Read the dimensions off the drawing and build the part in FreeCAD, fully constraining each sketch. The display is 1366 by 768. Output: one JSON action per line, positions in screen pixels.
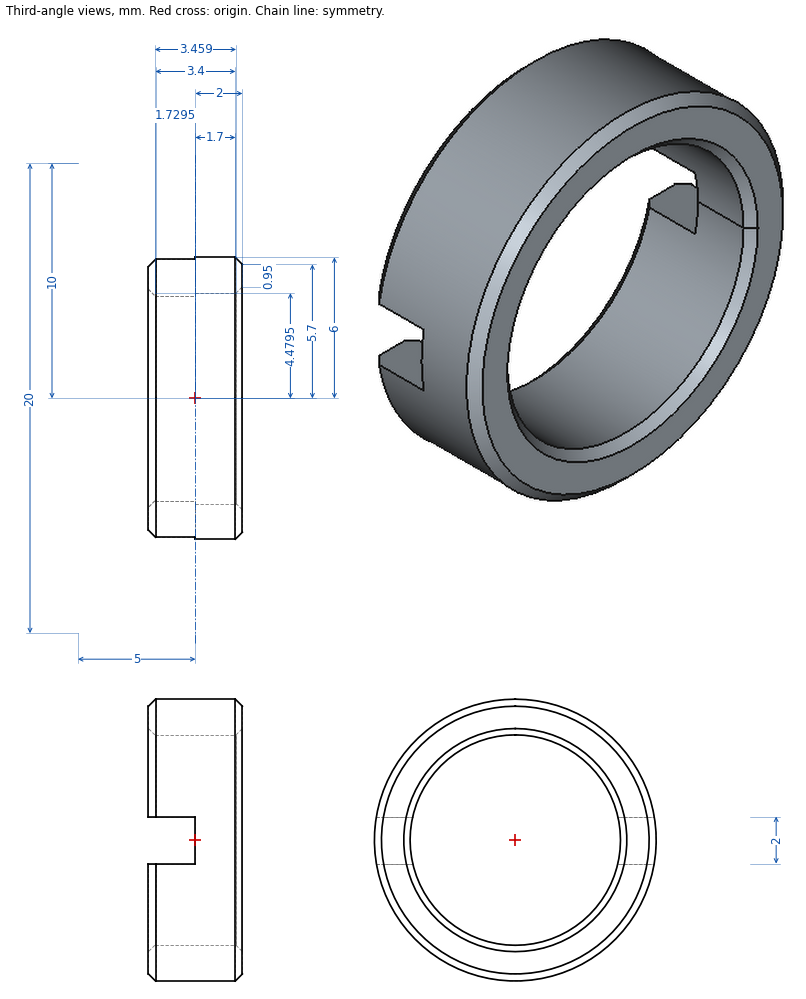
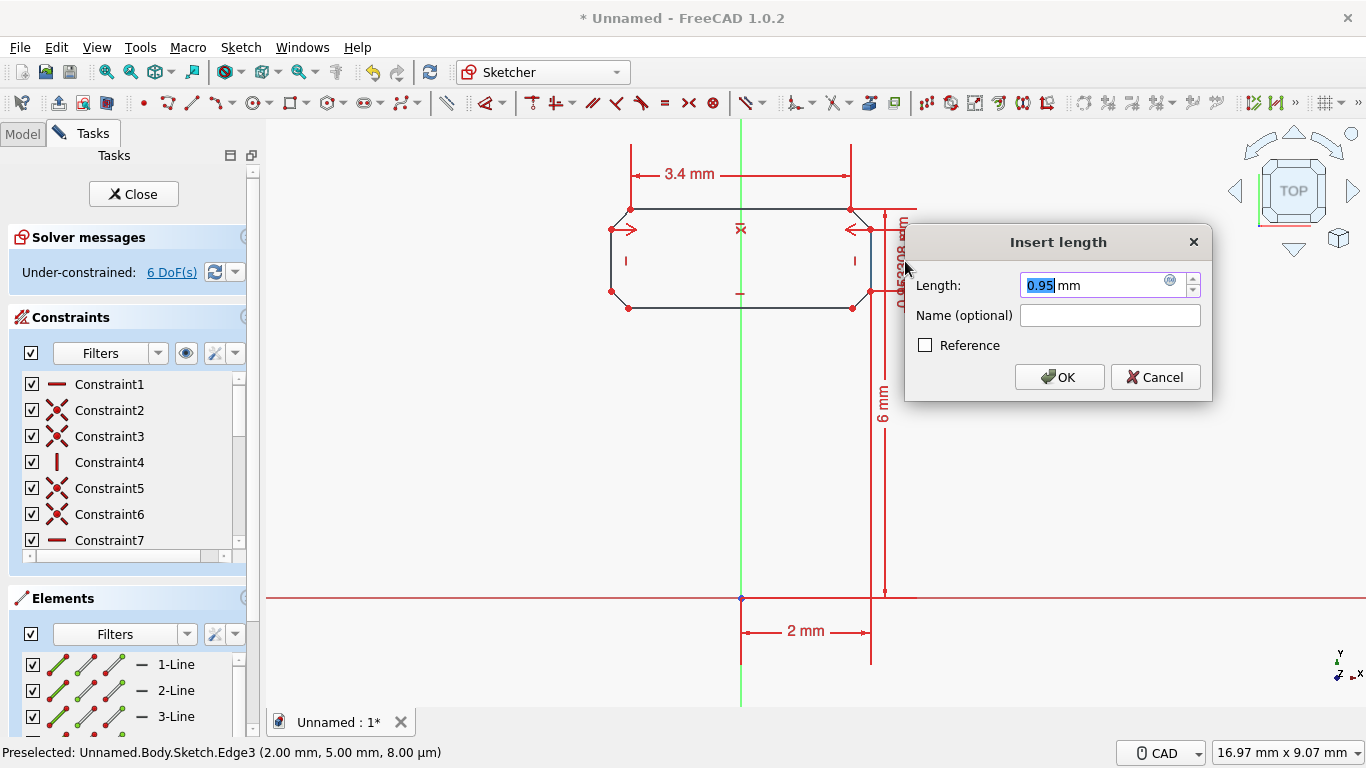
{"action": "type", "text": "0.95"}
{"action": "key", "text": "Return"}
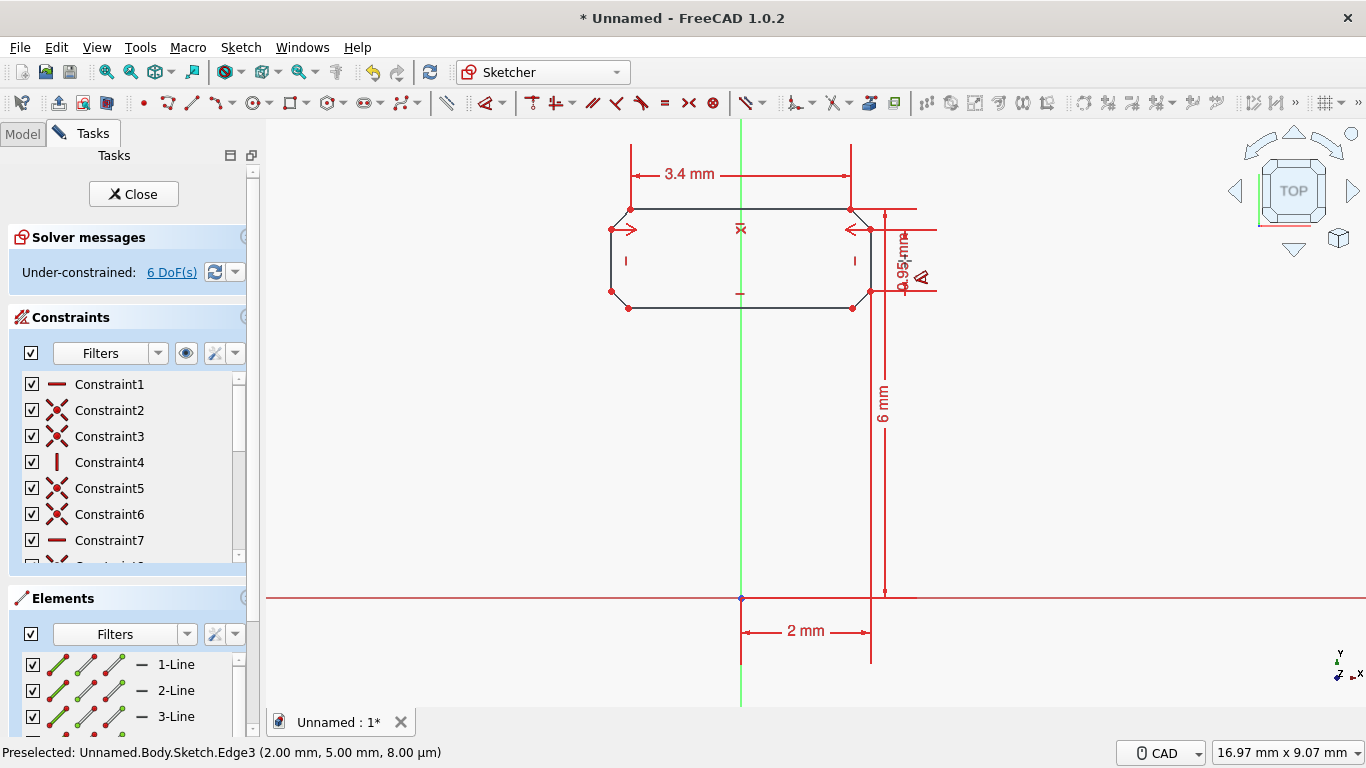
{"action": "left_click", "coordinate": [611, 248]}
{"action": "left_click", "coordinate": [577, 261]}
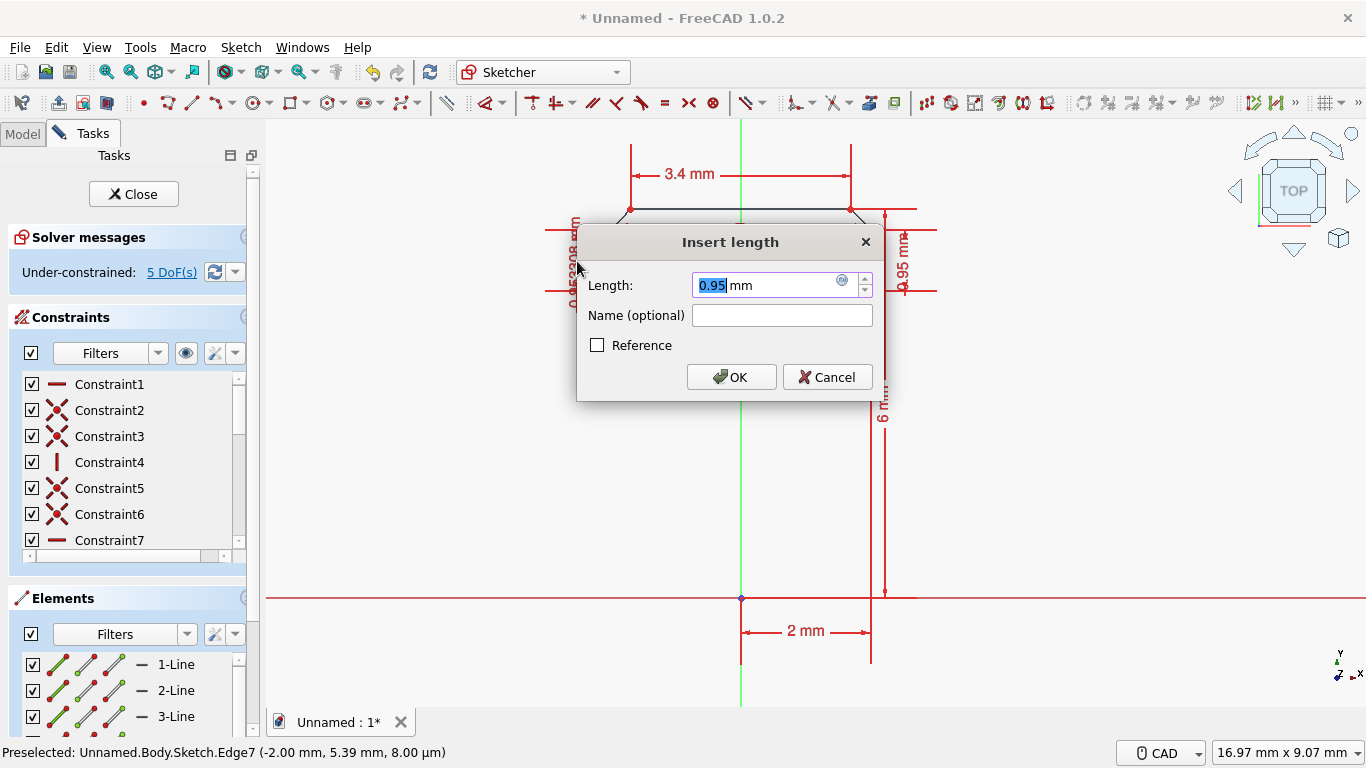
{"action": "type", "text": "0.95"}
{"action": "key", "text": "Return"}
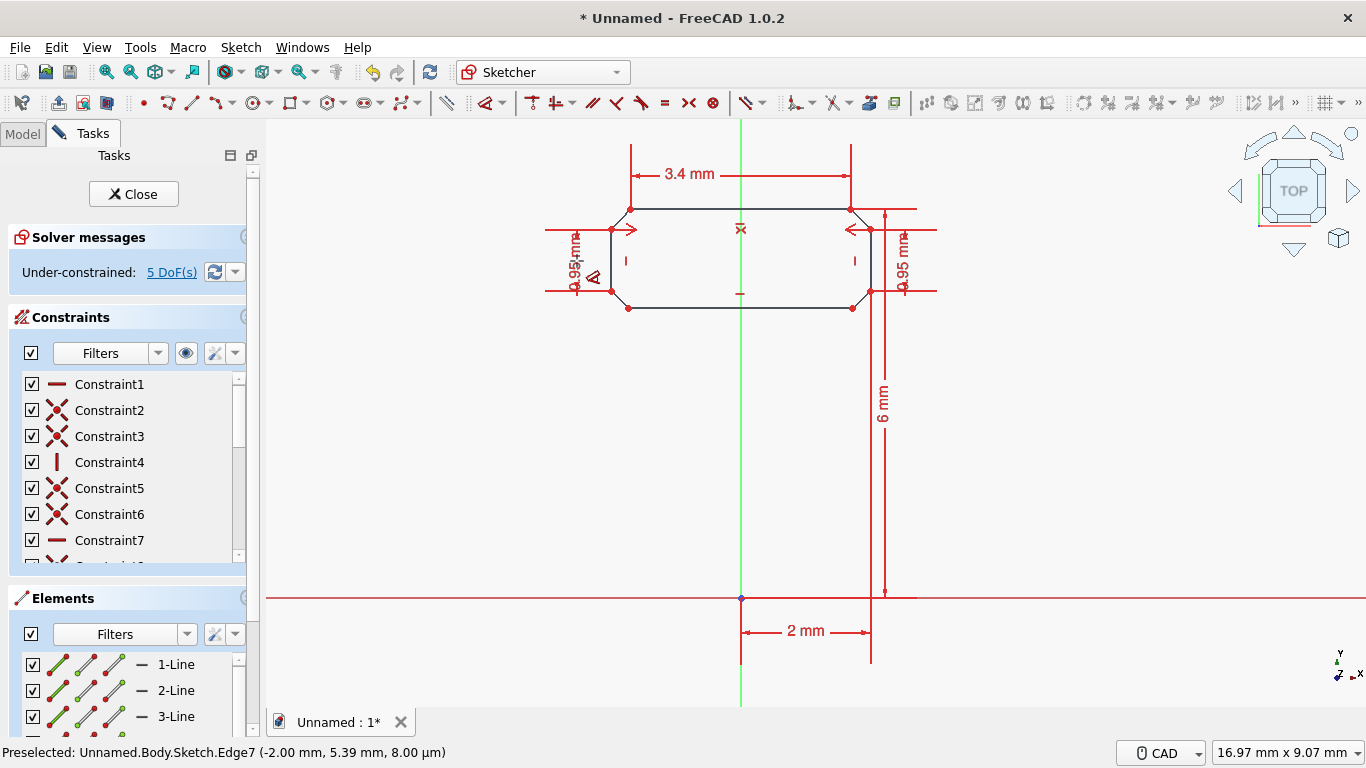
{"action": "left_click", "coordinate": [871, 230]}
{"action": "left_click", "coordinate": [905, 329]}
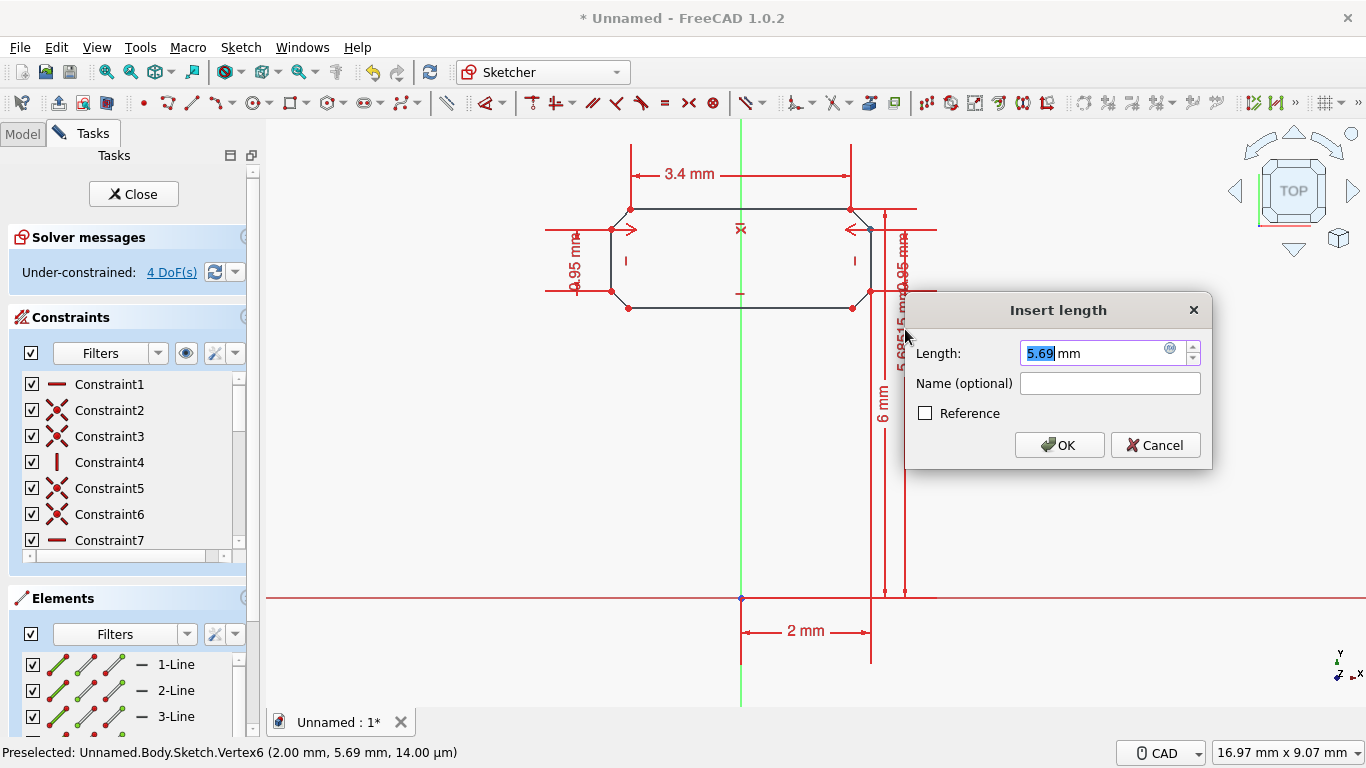
{"action": "type", "text": "5.7"}
{"action": "key", "text": "Return"}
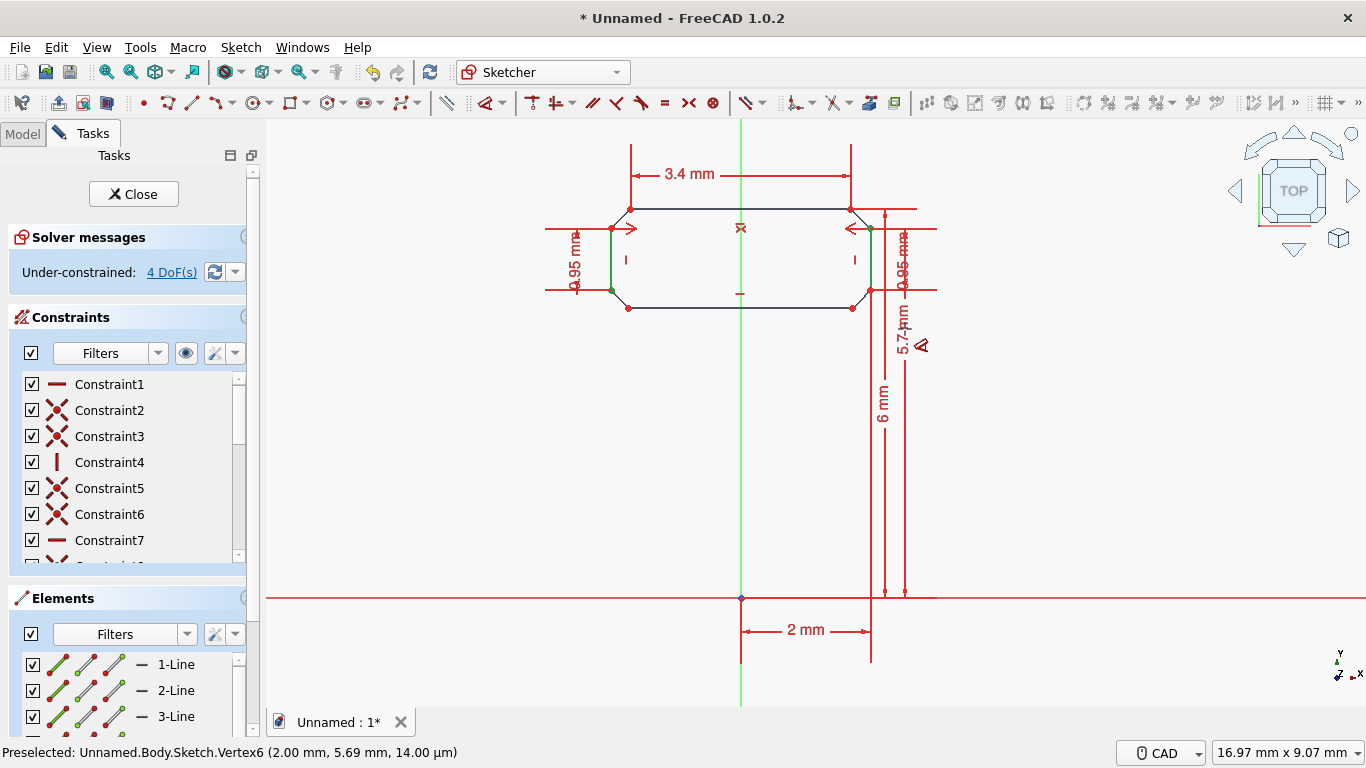
{"action": "left_click", "coordinate": [851, 209]}
{"action": "left_click", "coordinate": [796, 175]}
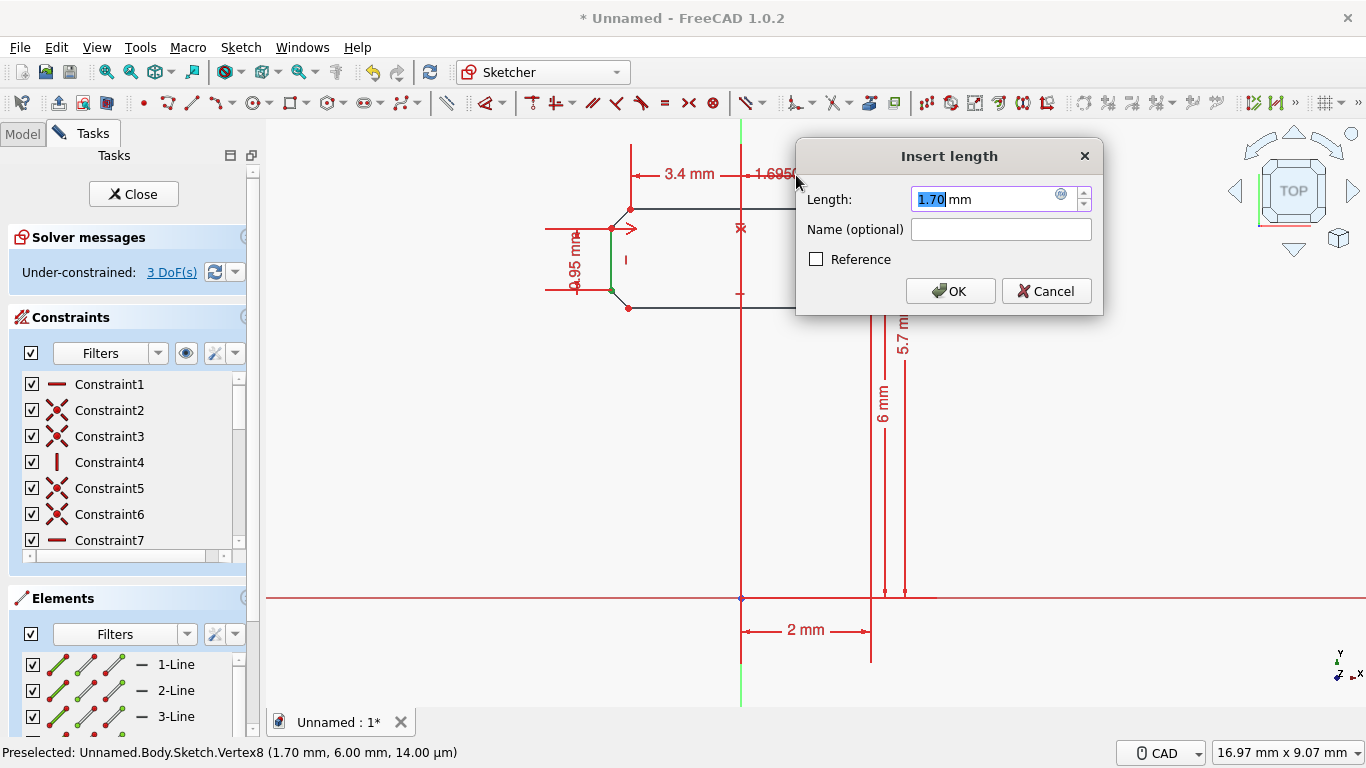
{"action": "type", "text": "1.7"}
{"action": "key", "text": "Return"}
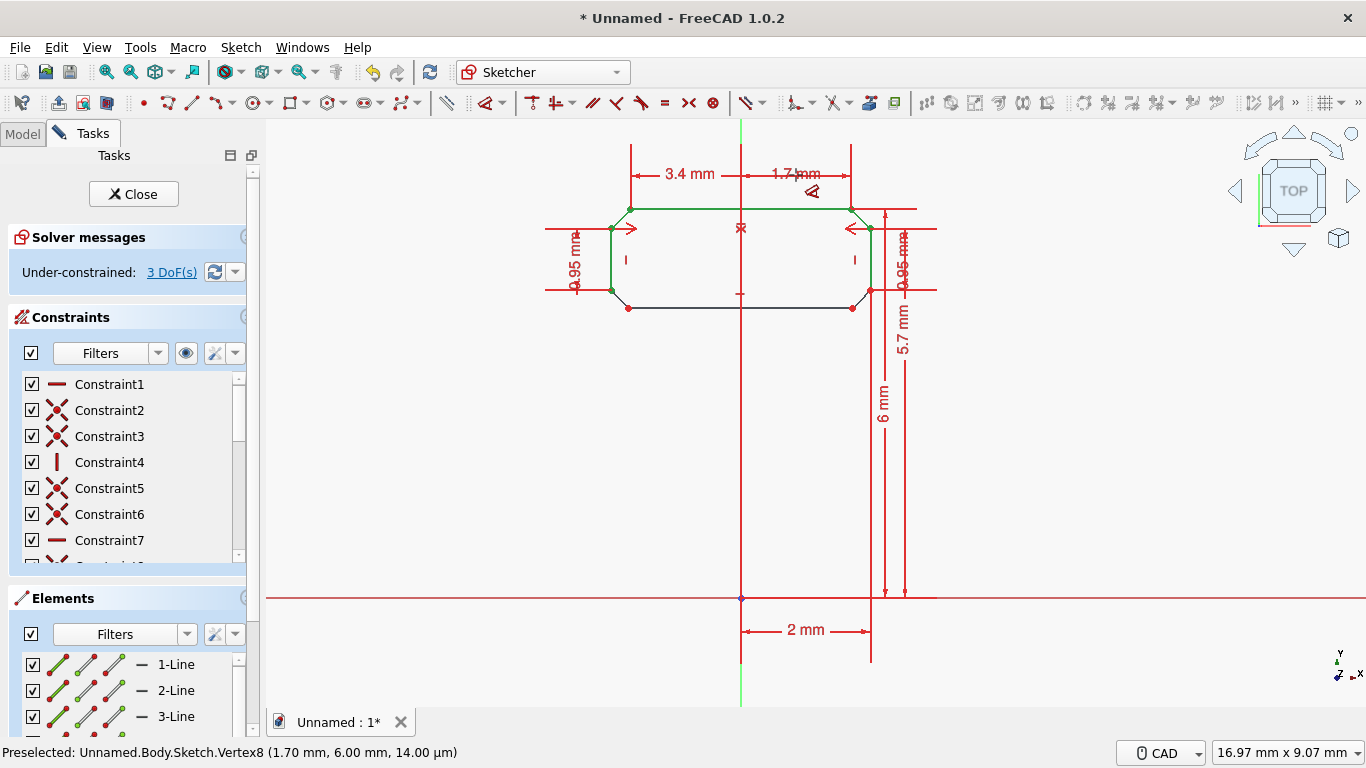
{"action": "left_click", "coordinate": [696, 308]}
{"action": "left_click", "coordinate": [689, 274]}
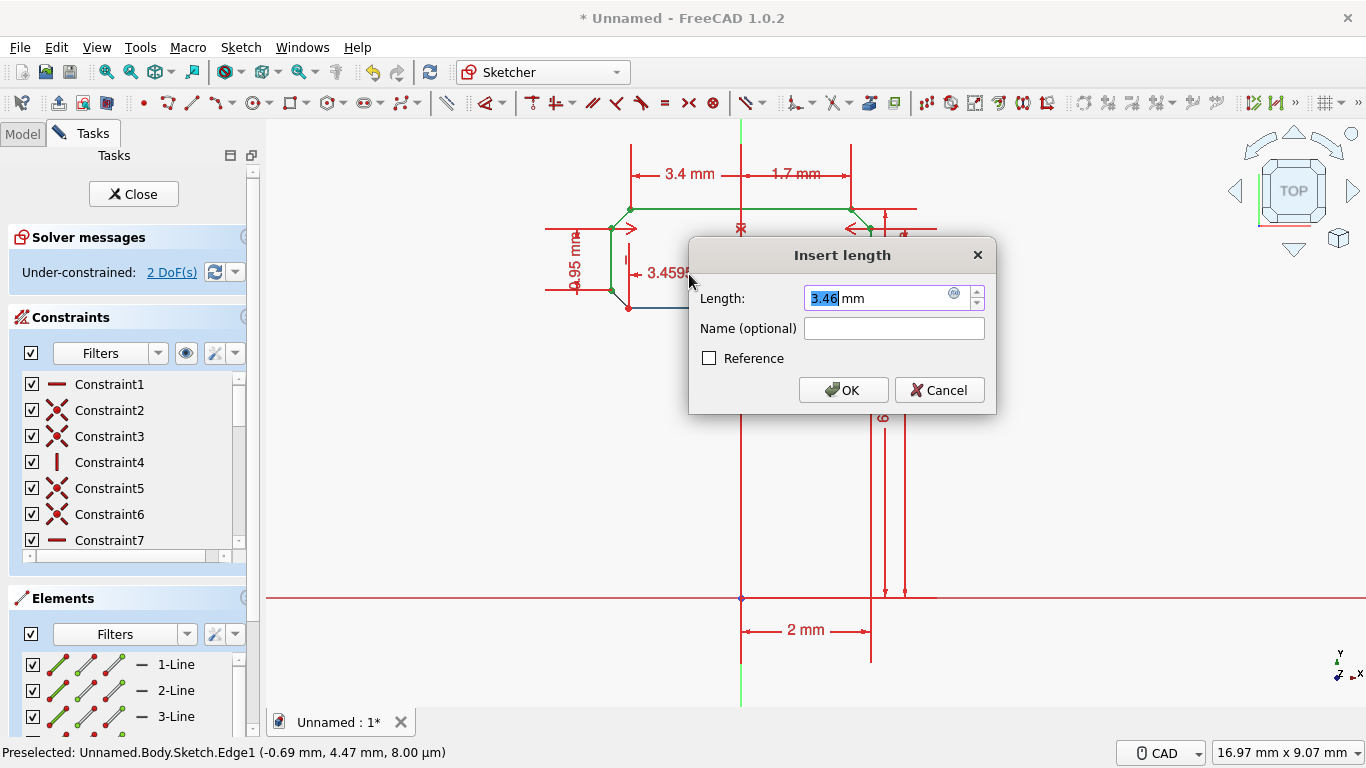
{"action": "type", "text": "3.459"}
{"action": "key", "text": "Return"}